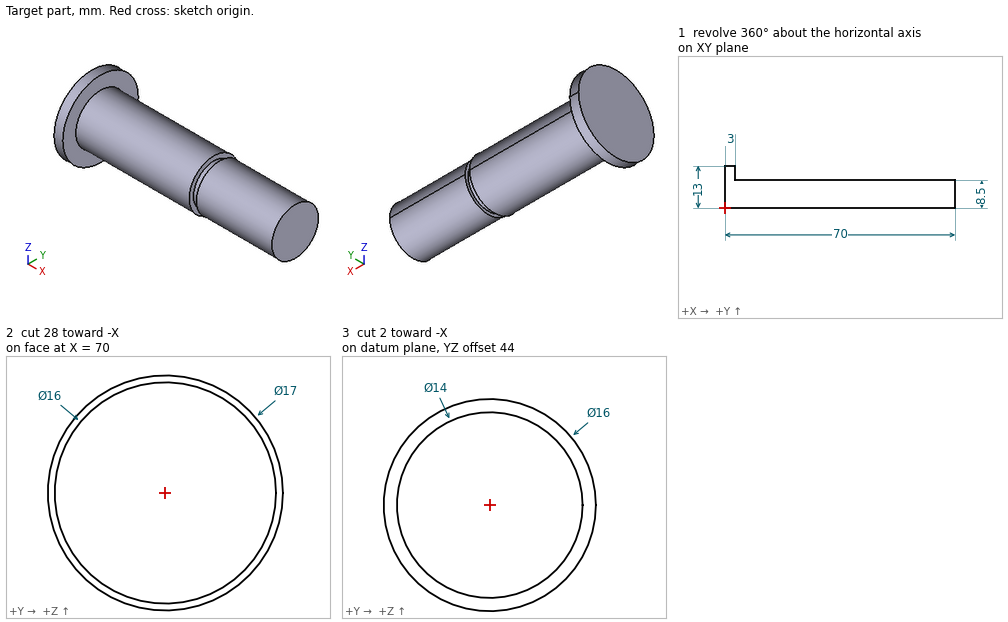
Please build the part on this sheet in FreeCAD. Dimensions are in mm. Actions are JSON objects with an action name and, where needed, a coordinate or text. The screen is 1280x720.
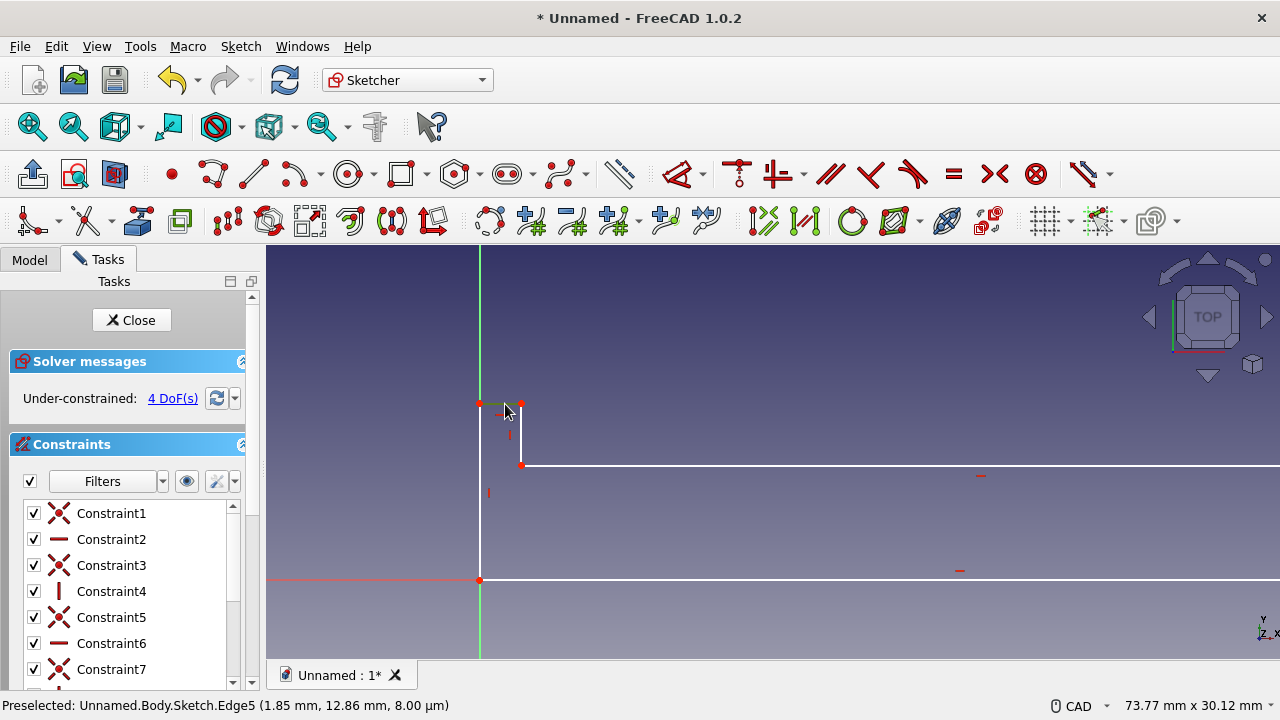
{"action": "key", "text": "l"}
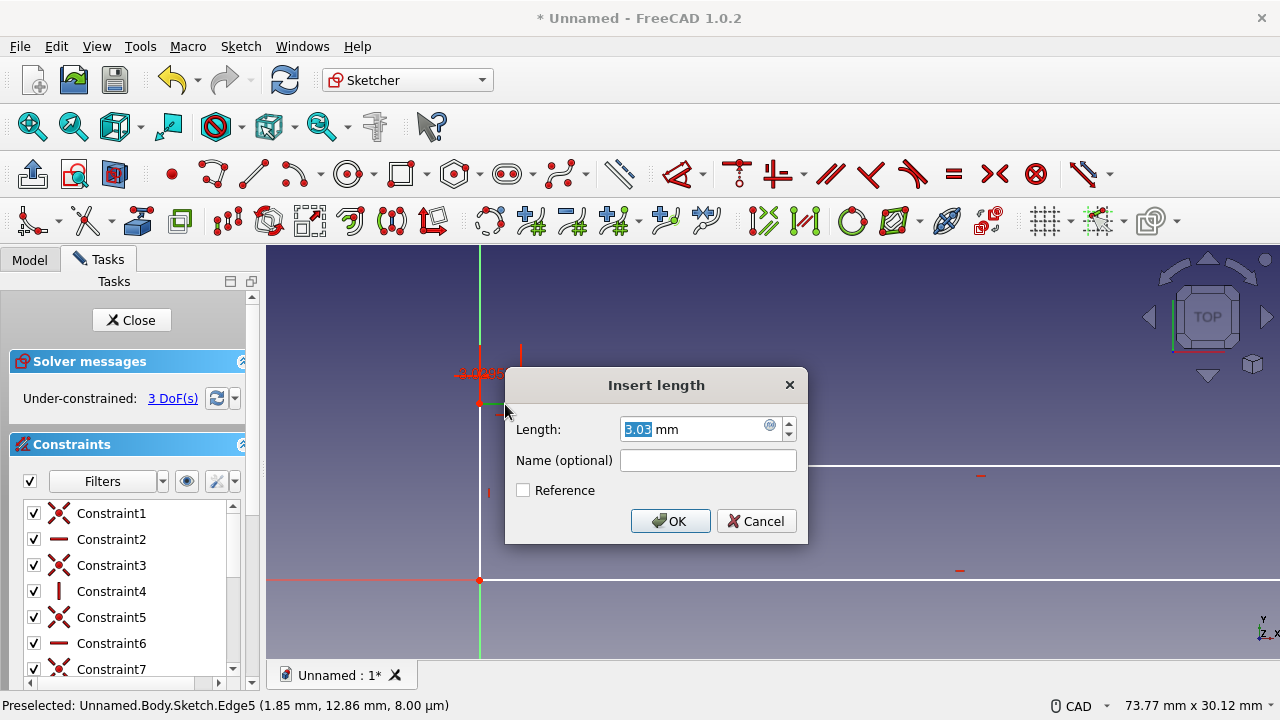
{"action": "type", "text": "3"}
{"action": "key", "text": "Return"}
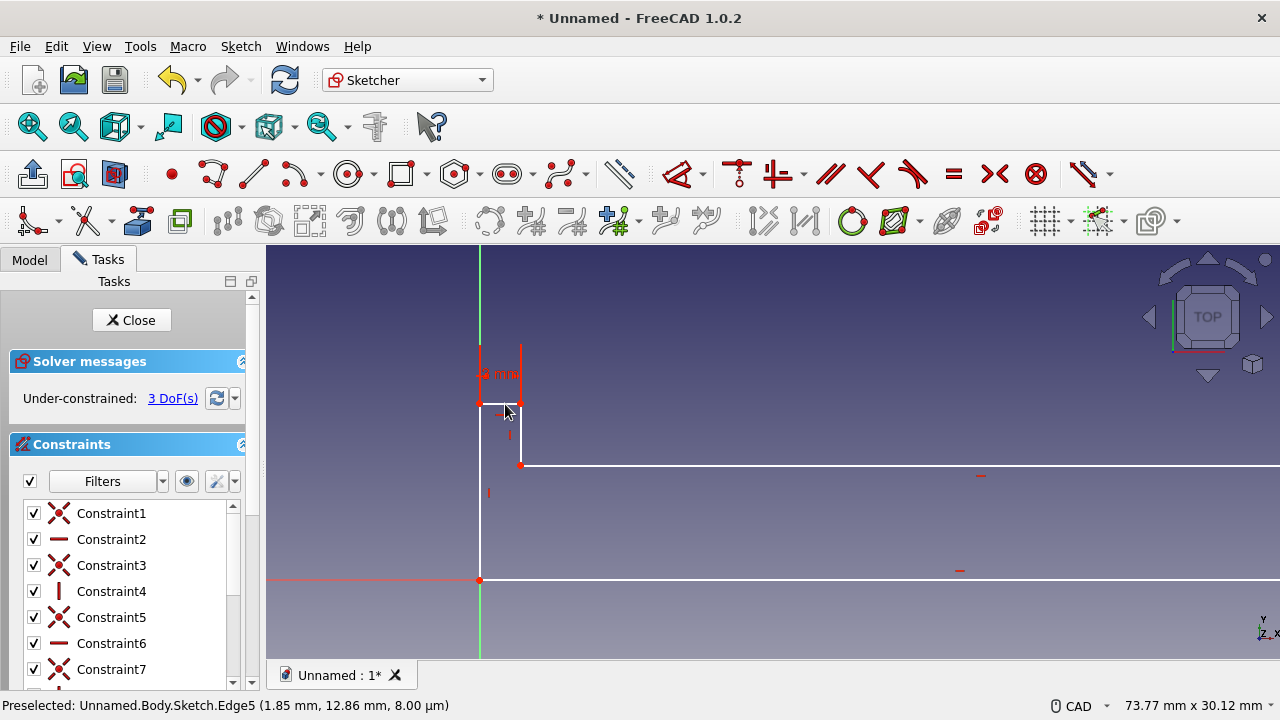
{"action": "left_click", "coordinate": [768, 580]}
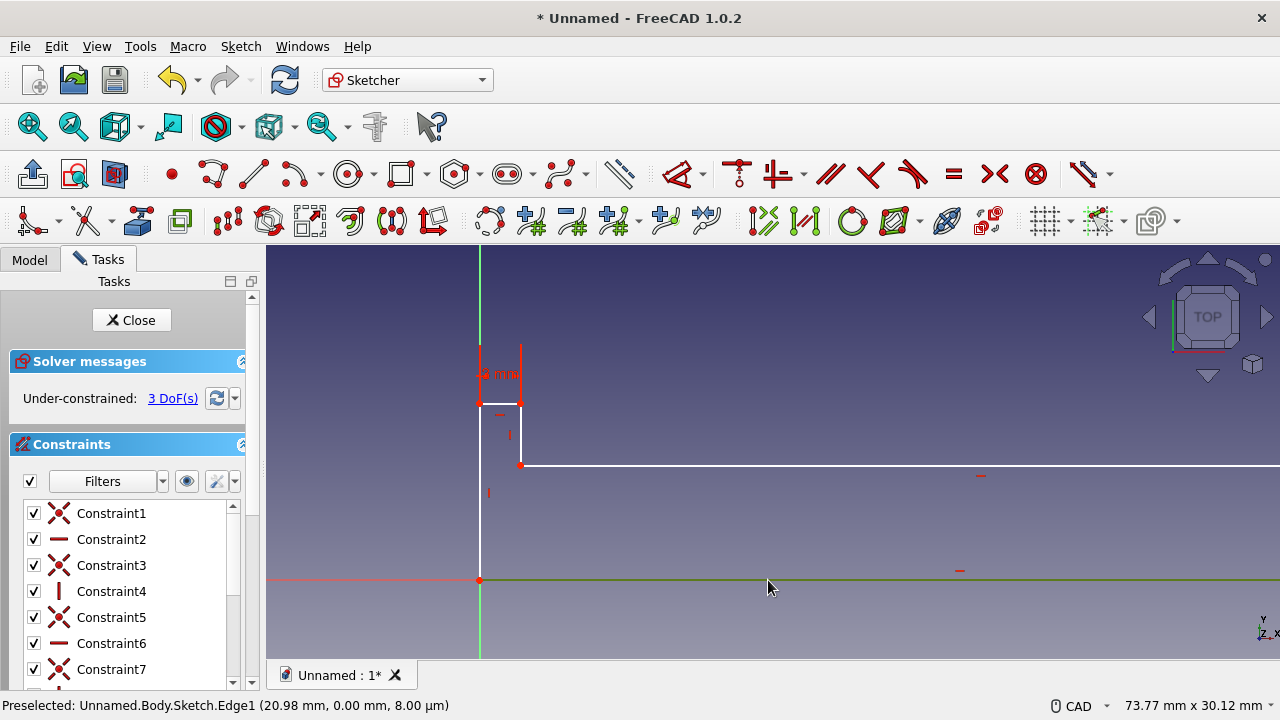
{"action": "key", "text": "l"}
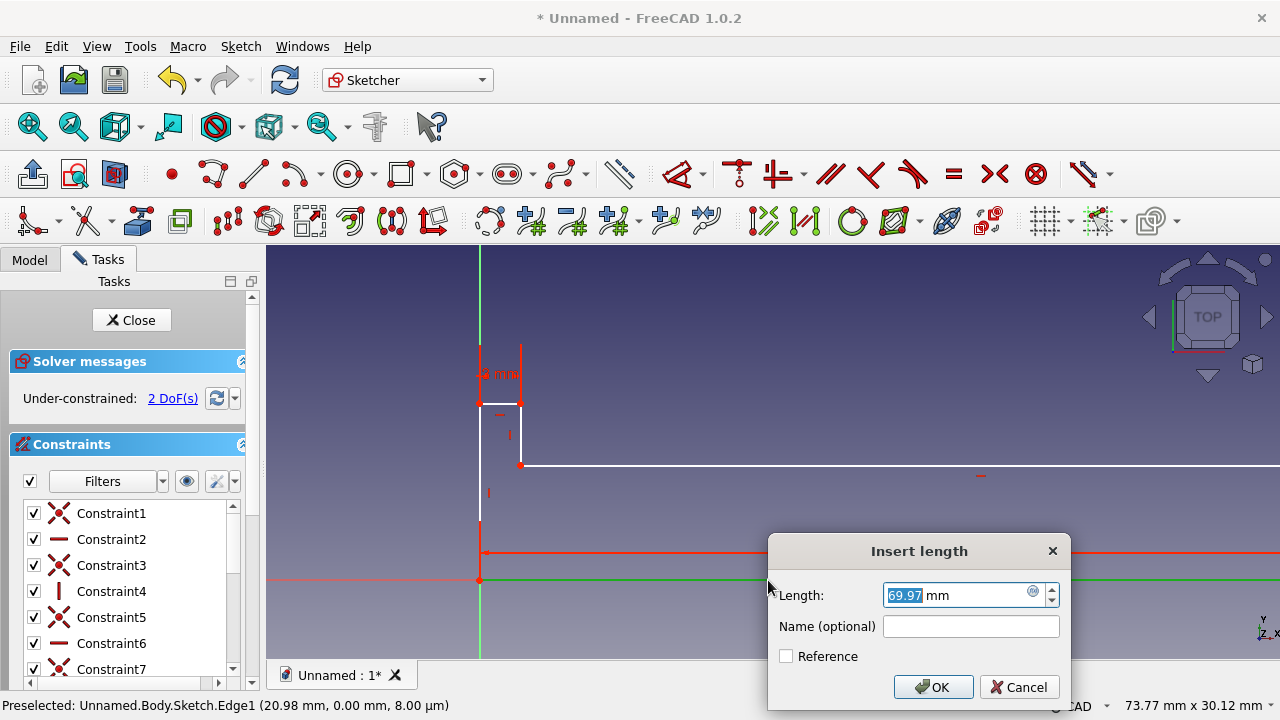
{"action": "type", "text": "70"}
{"action": "key", "text": "Return"}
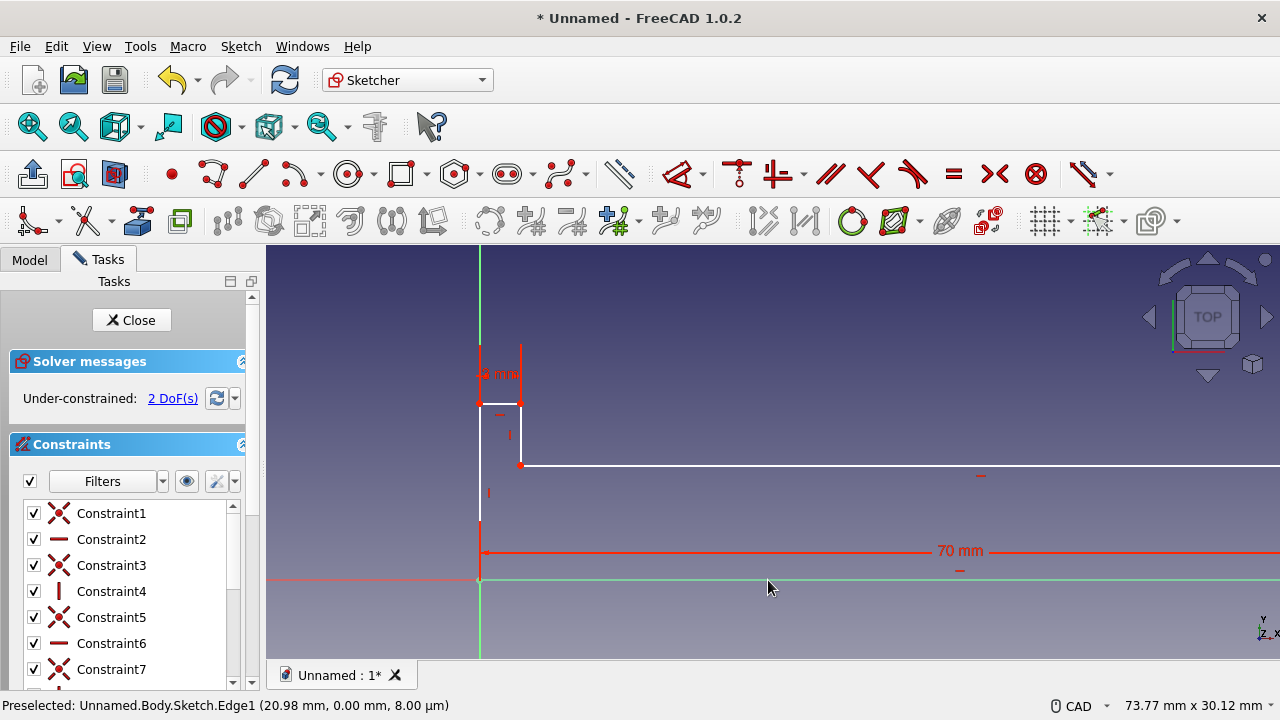
{"action": "left_click", "coordinate": [480, 457]}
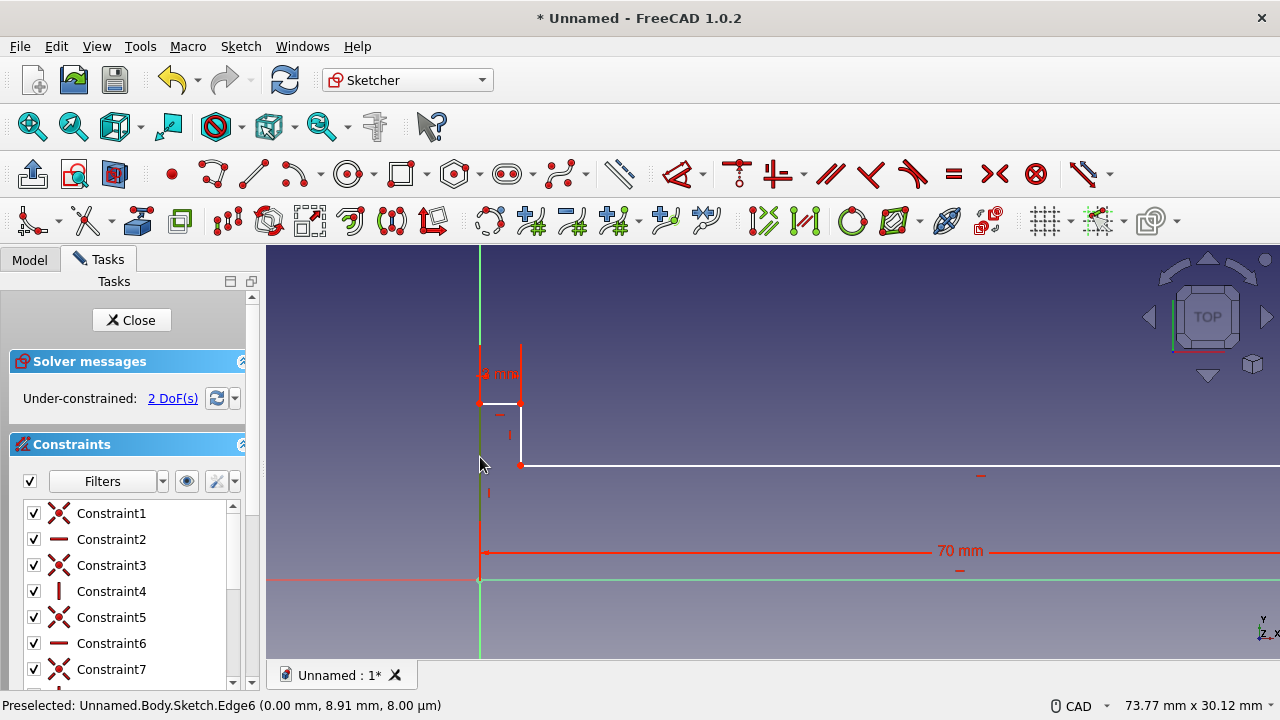
{"action": "left_click", "coordinate": [702, 174]}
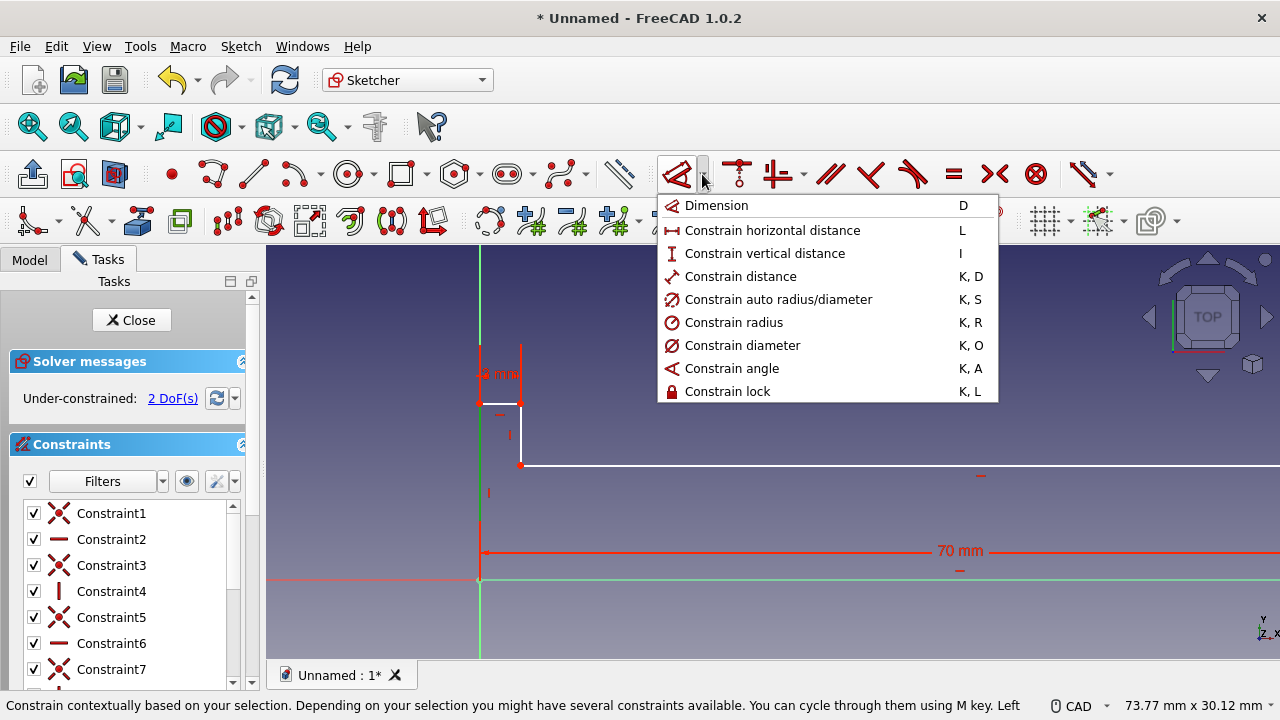
{"action": "left_click", "coordinate": [828, 254]}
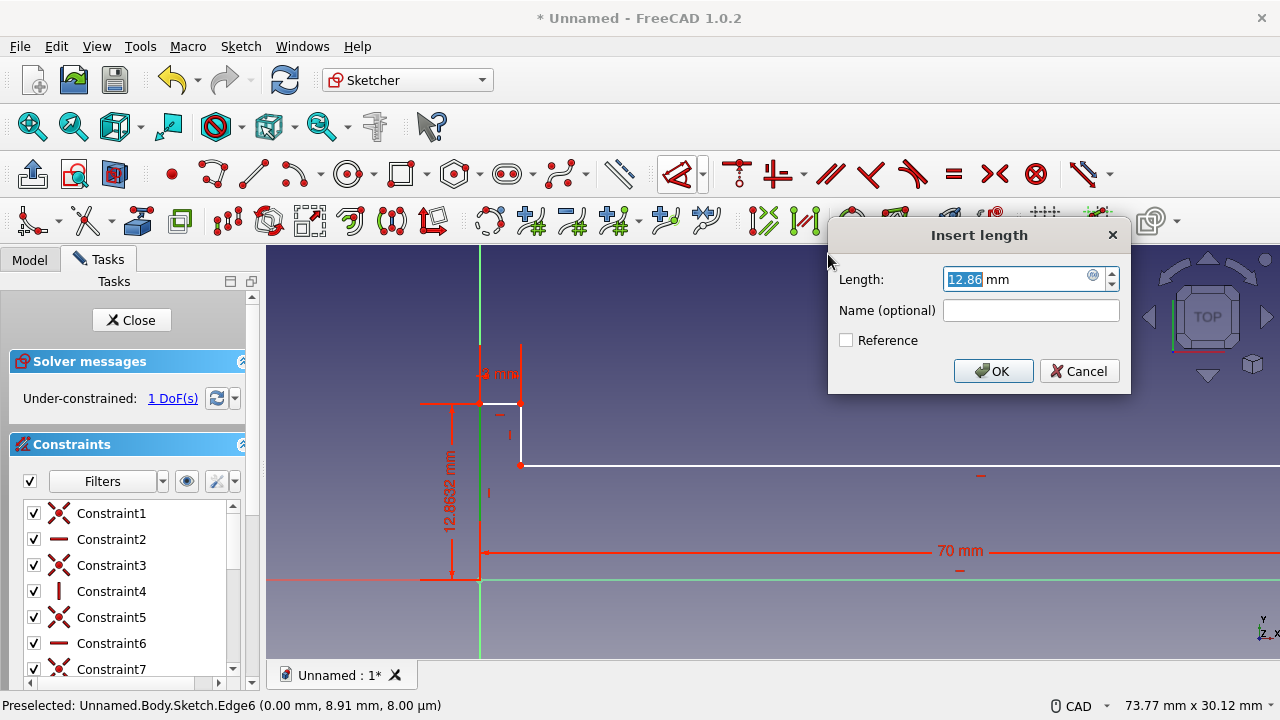
{"action": "type", "text": "13"}
{"action": "key", "text": "Return"}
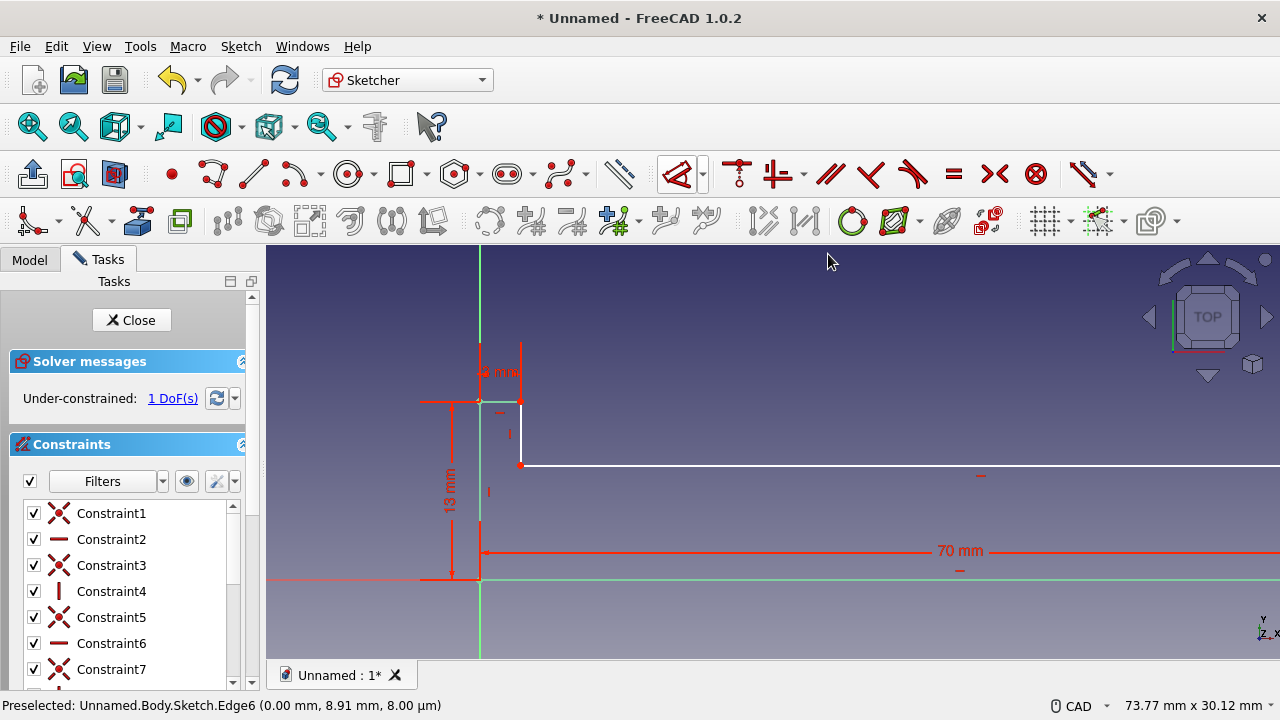
{"action": "scroll", "coordinate": [393, 404], "scroll_direction": "down", "scroll_amount": 3}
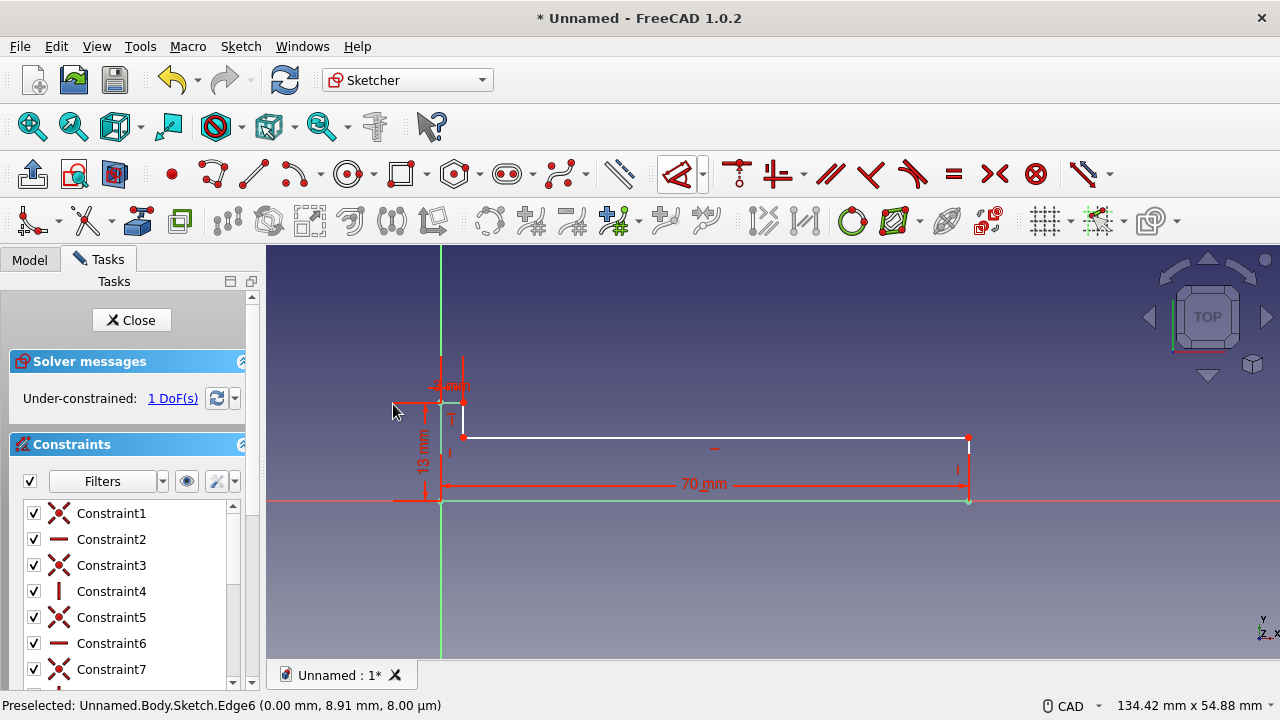
{"action": "left_click", "coordinate": [969, 482]}